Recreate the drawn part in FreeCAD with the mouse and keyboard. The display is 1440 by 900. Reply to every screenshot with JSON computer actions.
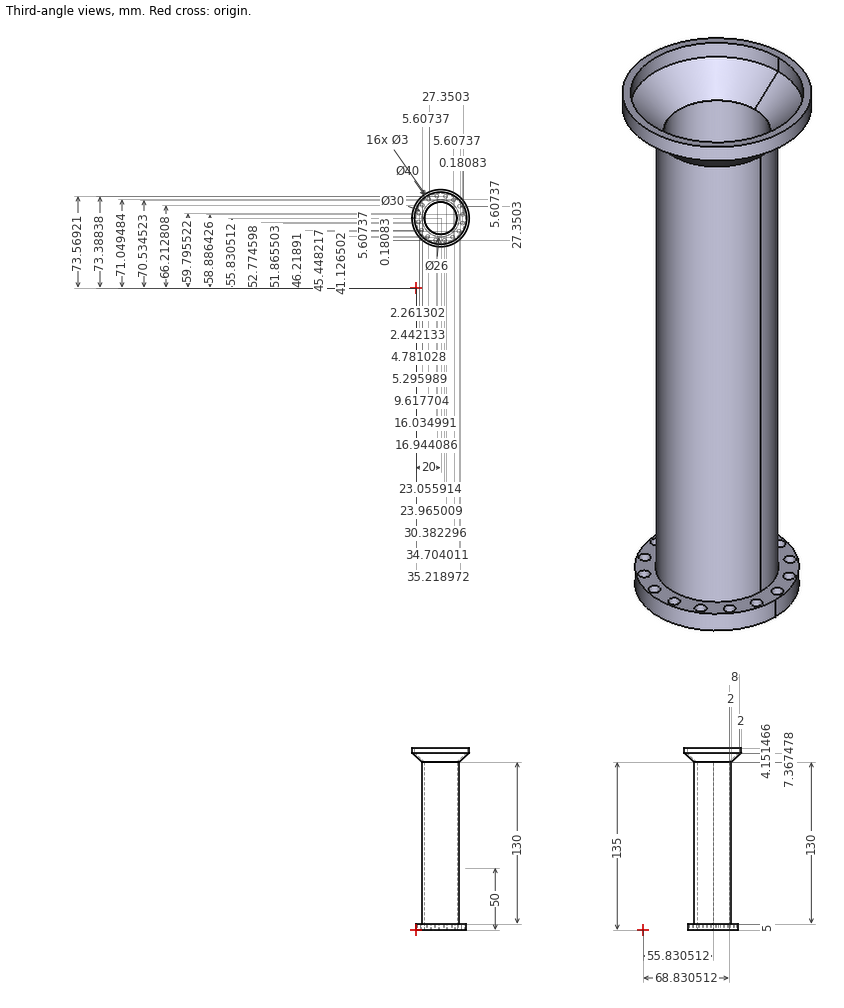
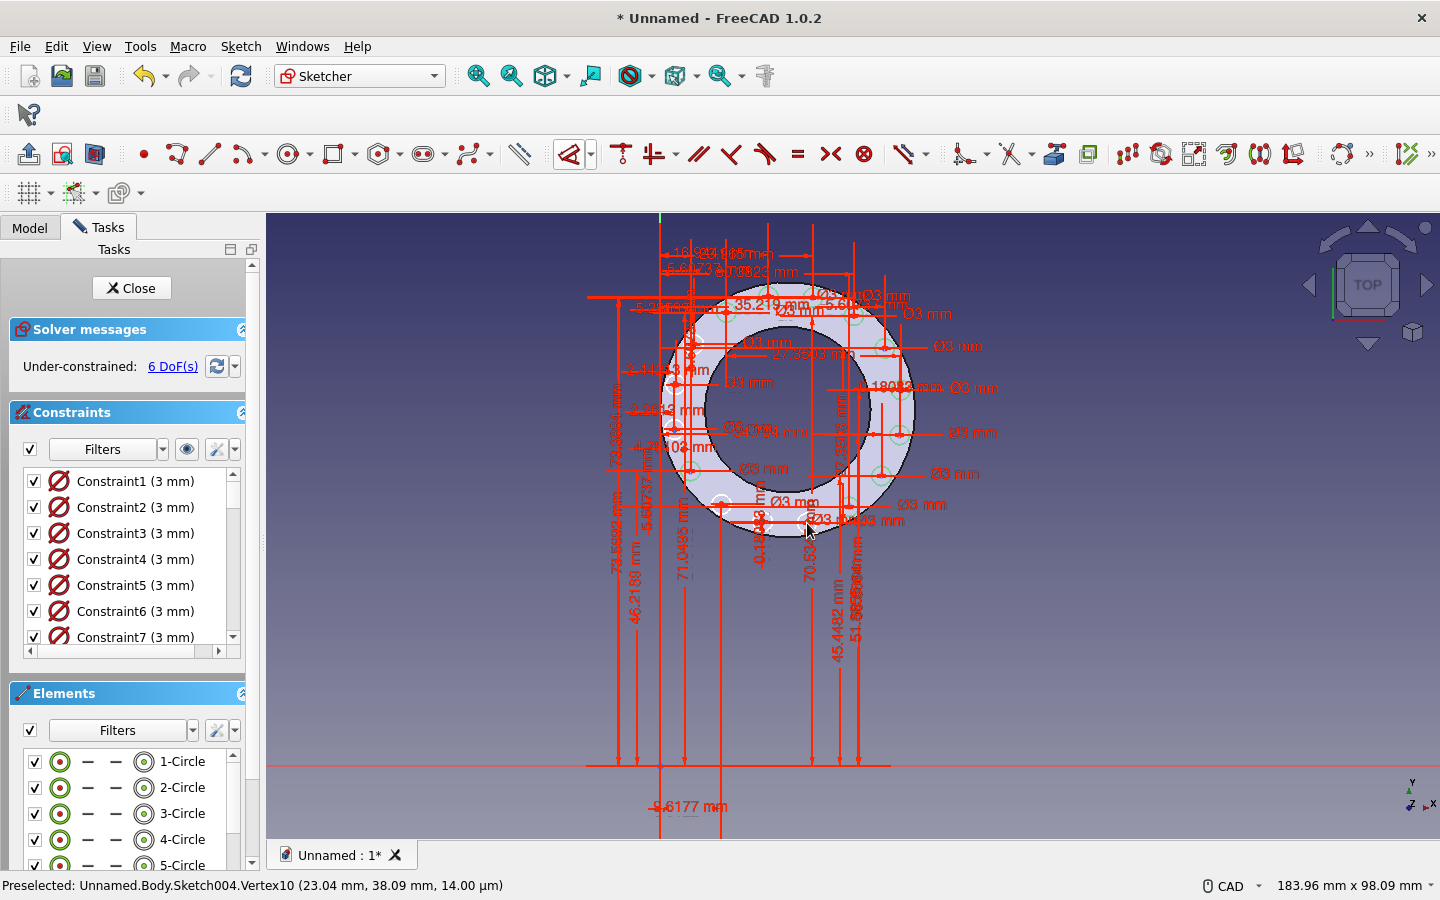
{"action": "key", "text": "l"}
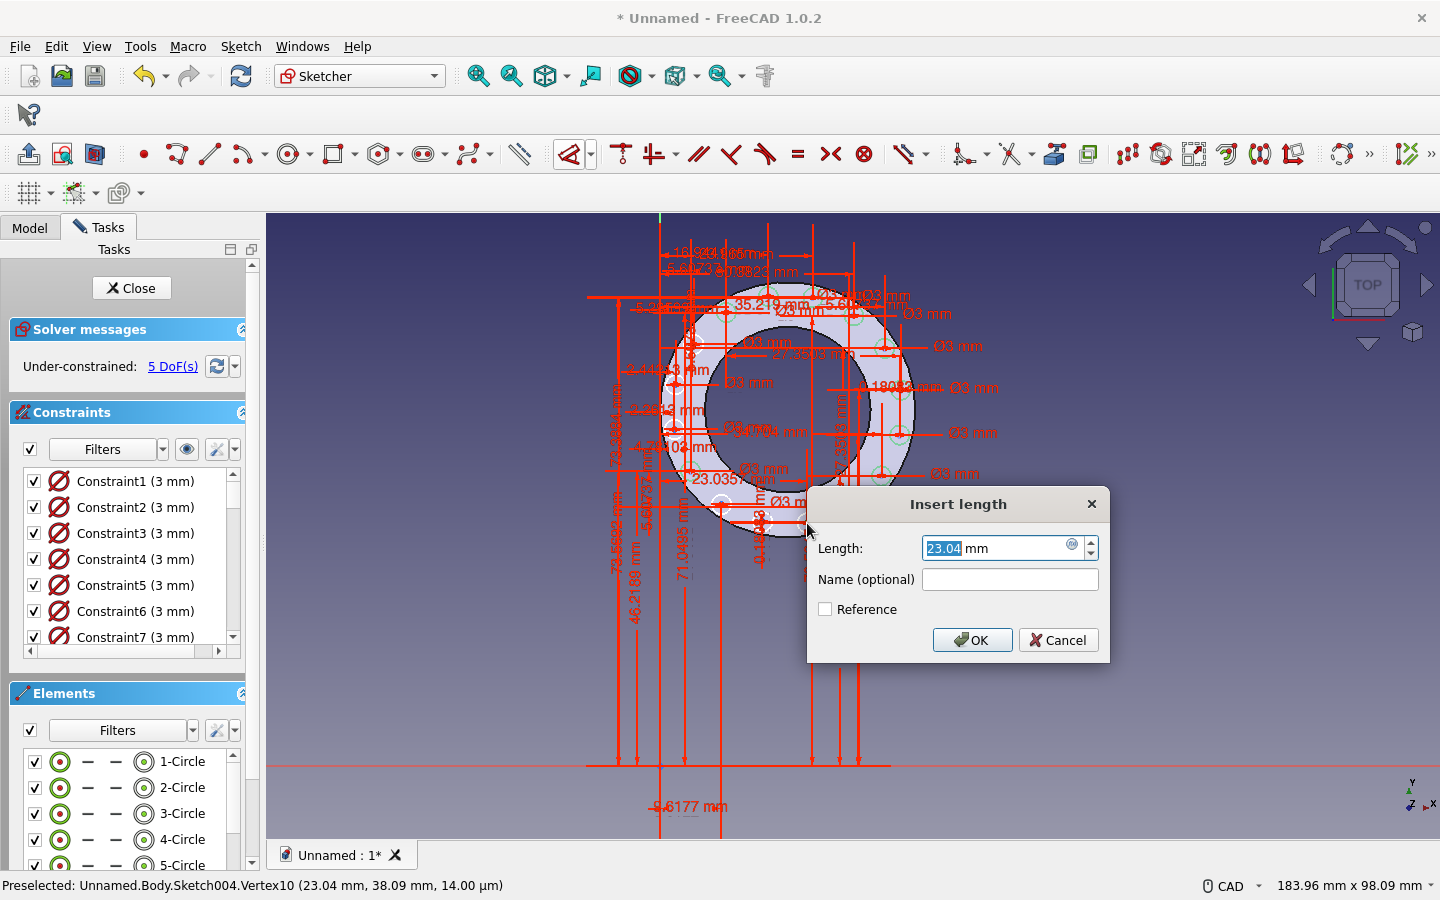
{"action": "type", "text": "23.055914"}
{"action": "key", "text": "Return"}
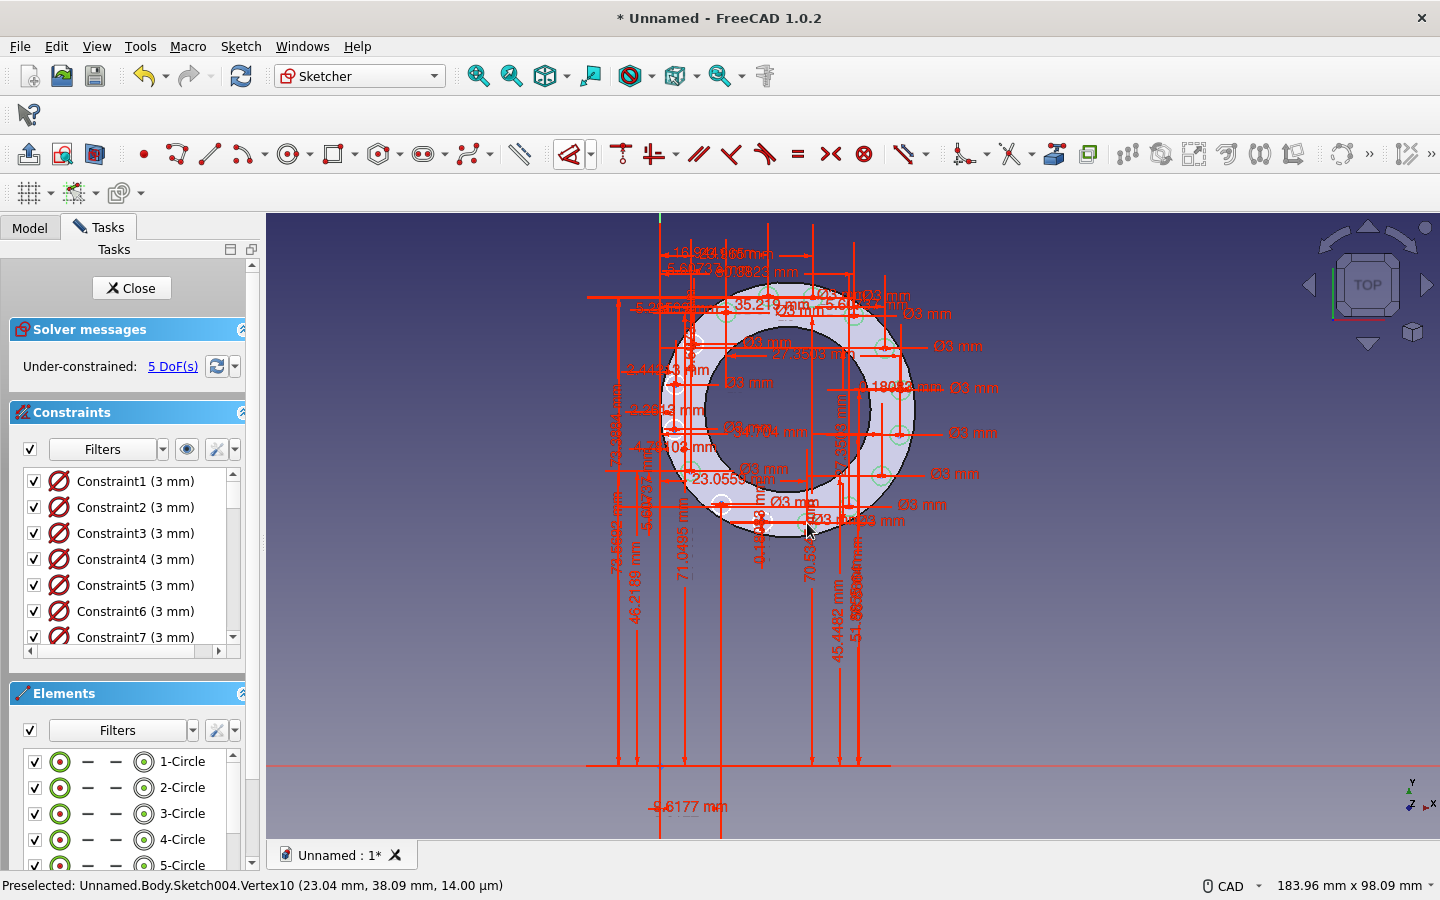
{"action": "left_click", "coordinate": [763, 522]}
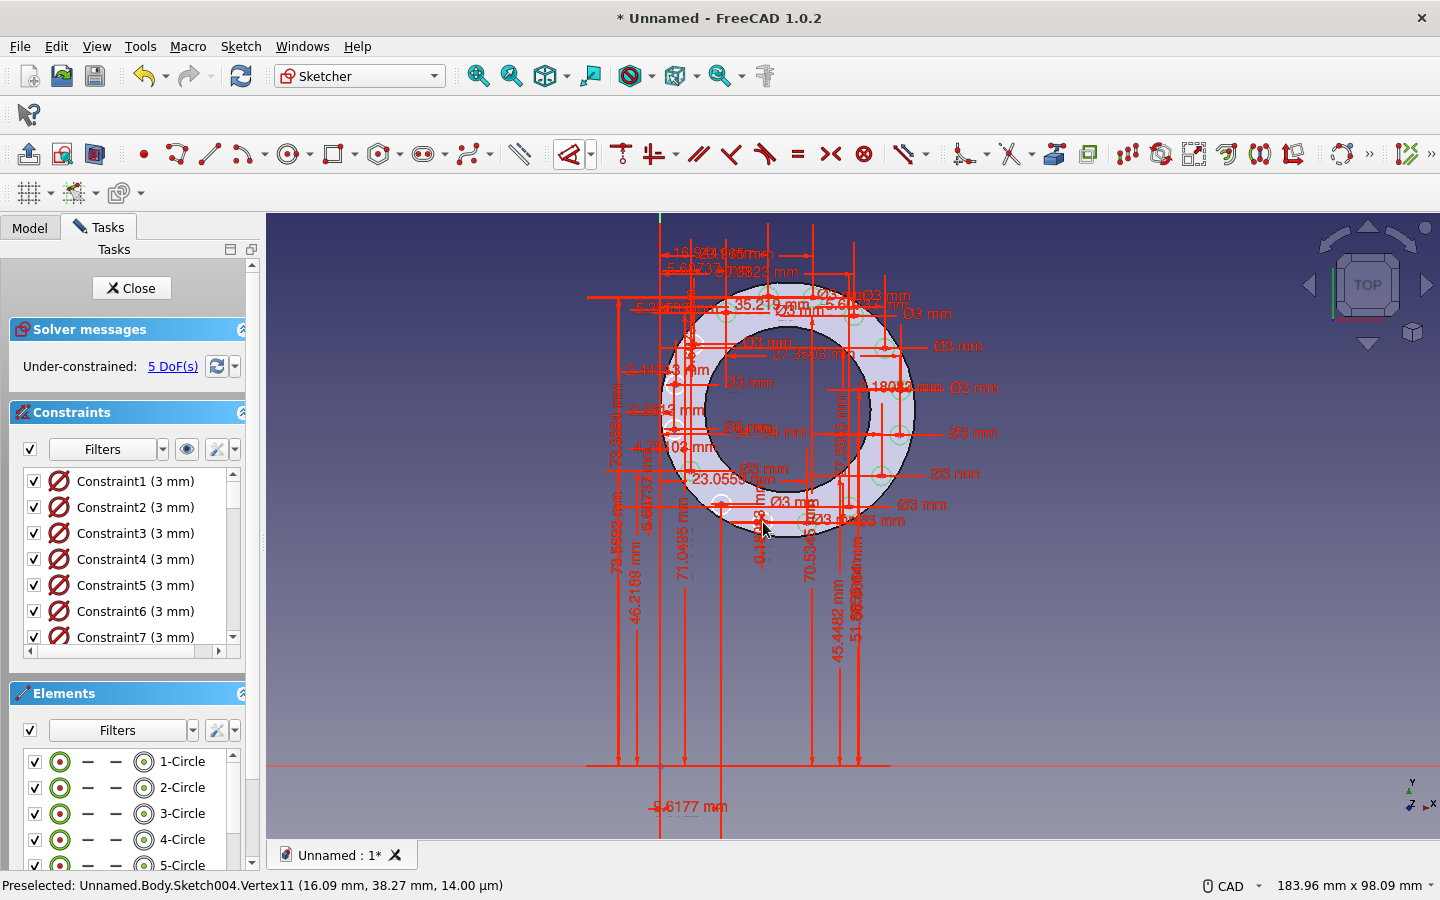
{"action": "key", "text": "l"}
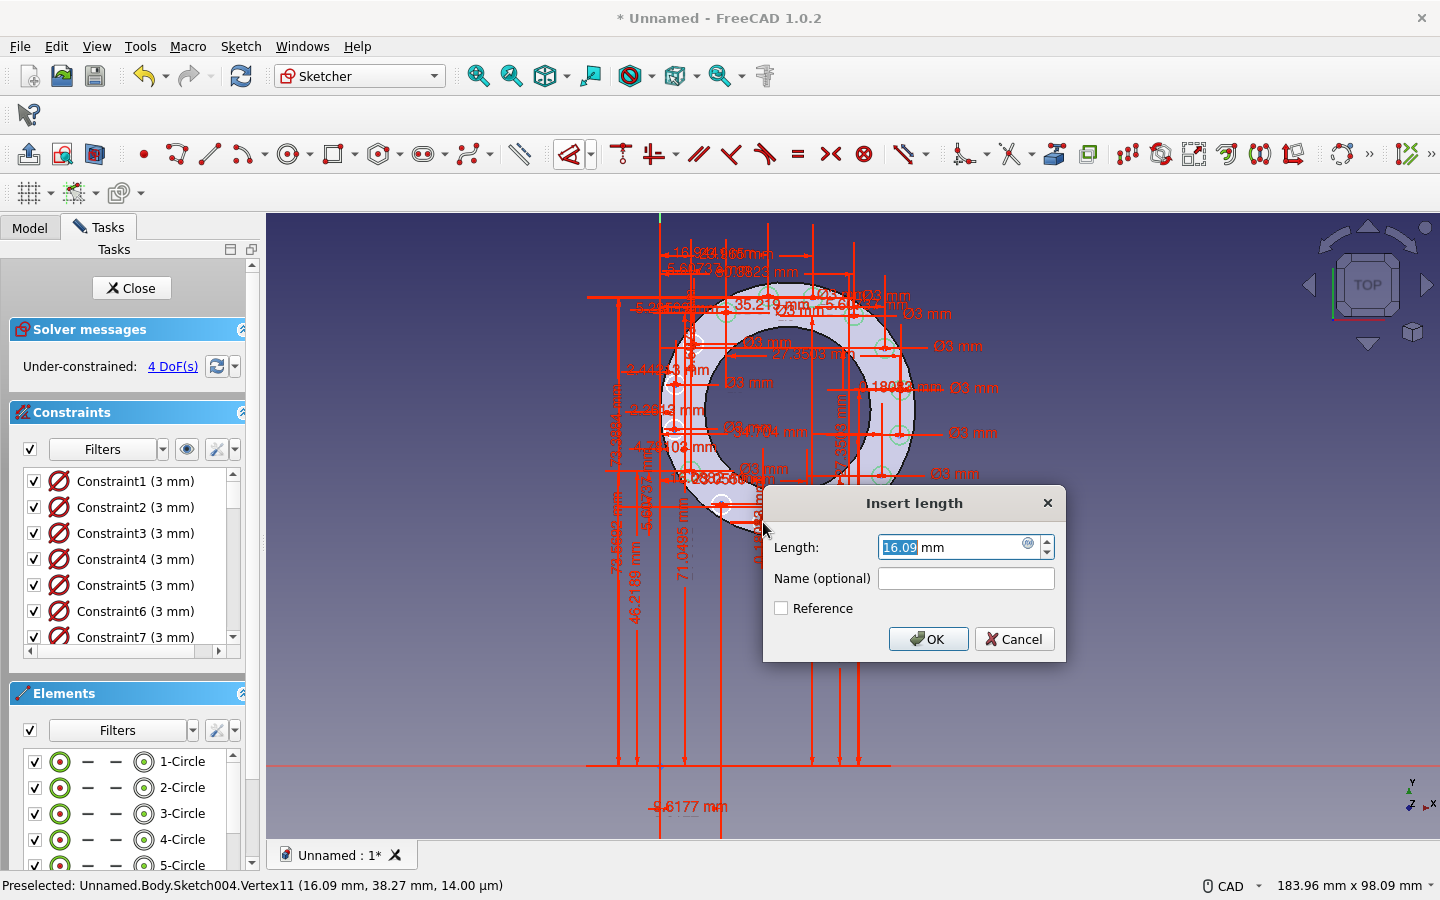
{"action": "type", "text": "16.034991"}
{"action": "key", "text": "Return"}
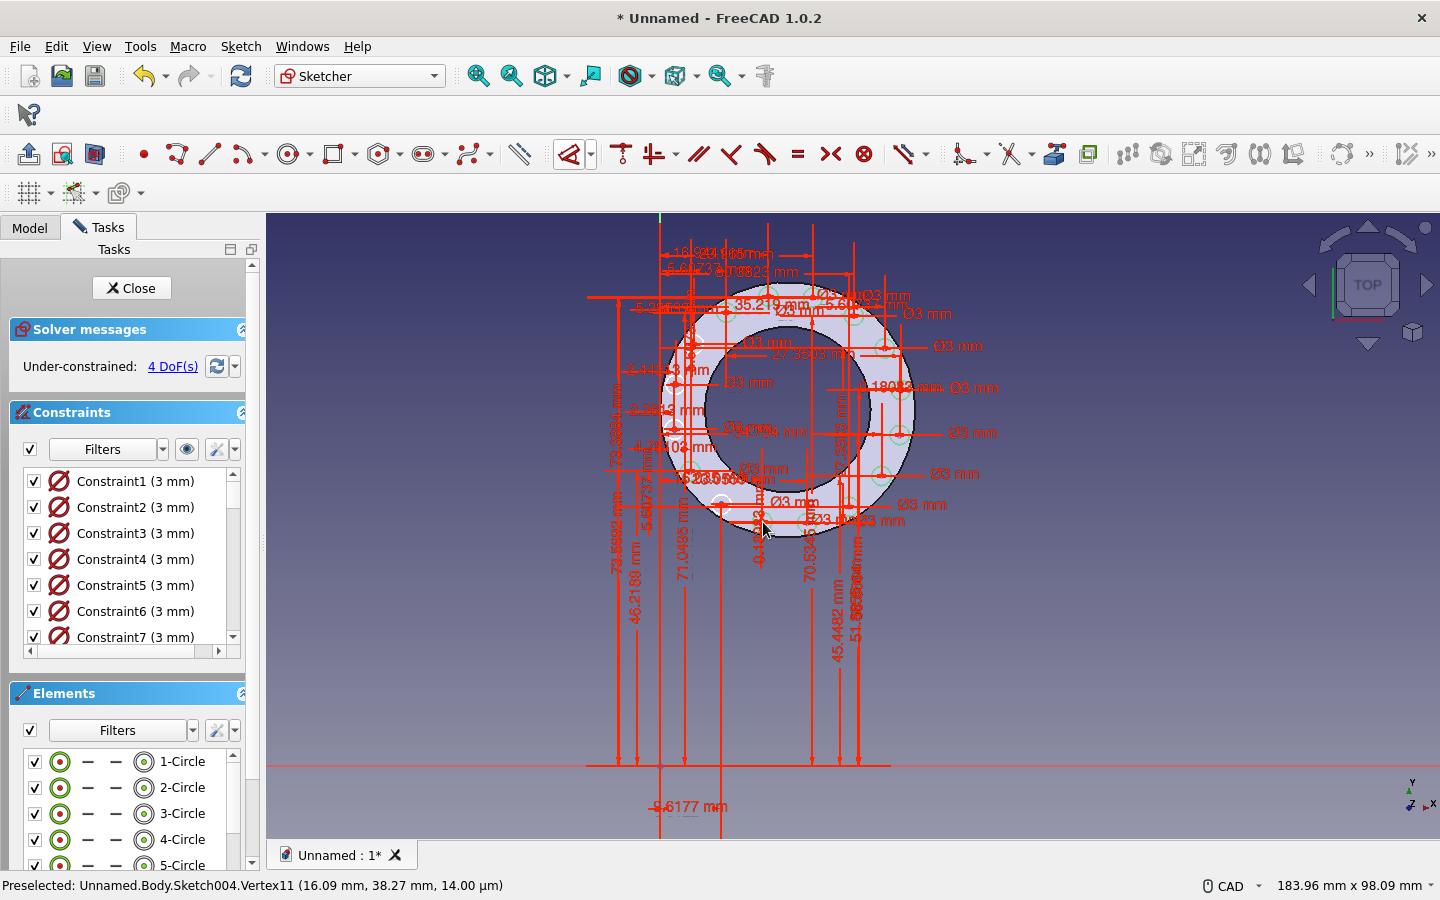
{"action": "left_click", "coordinate": [721, 504]}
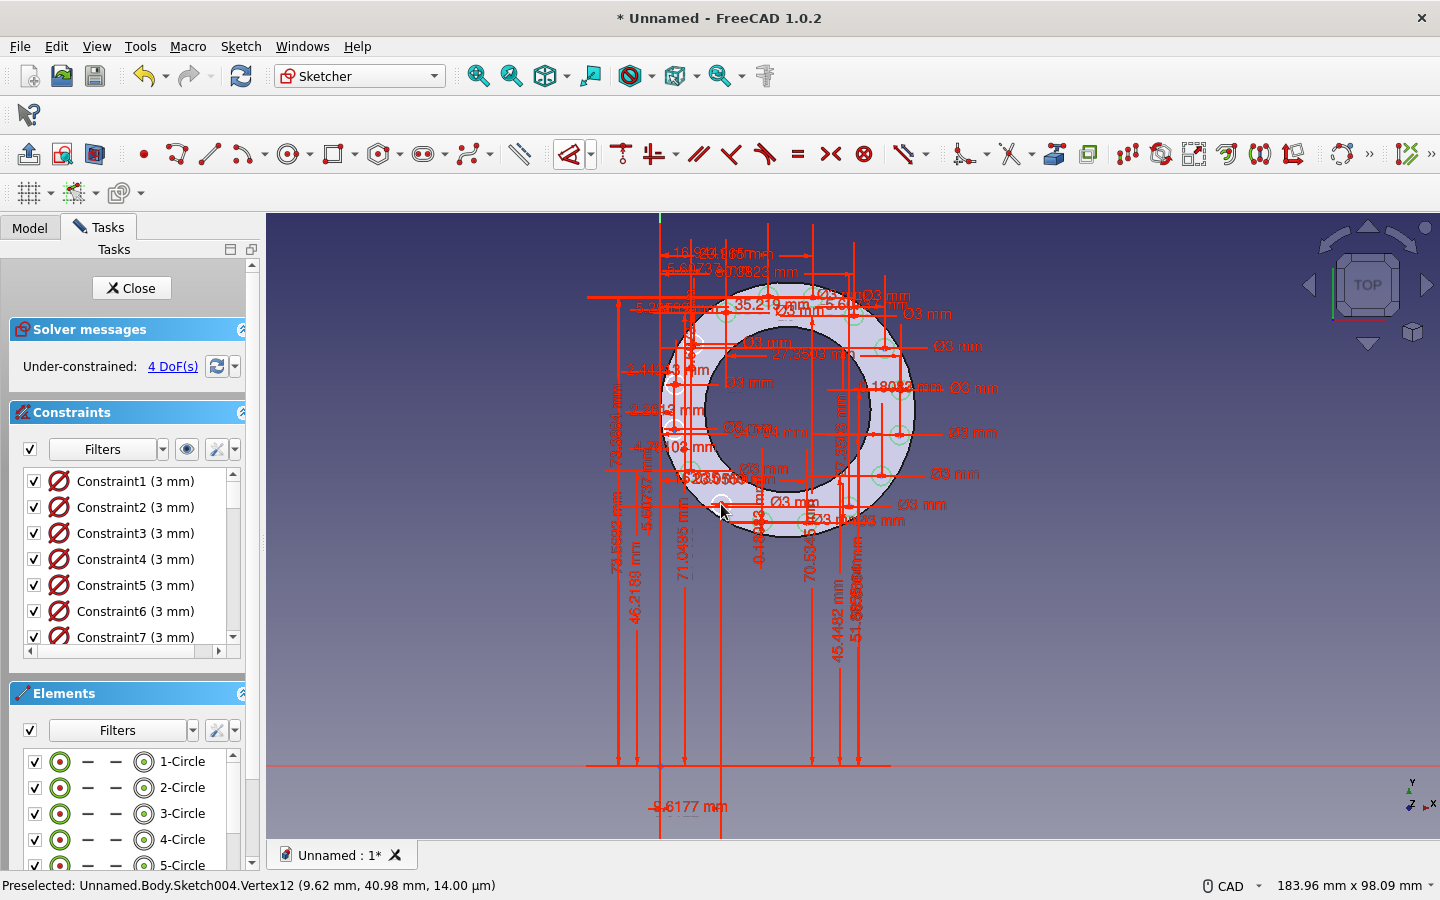
{"action": "left_click", "coordinate": [590, 154]}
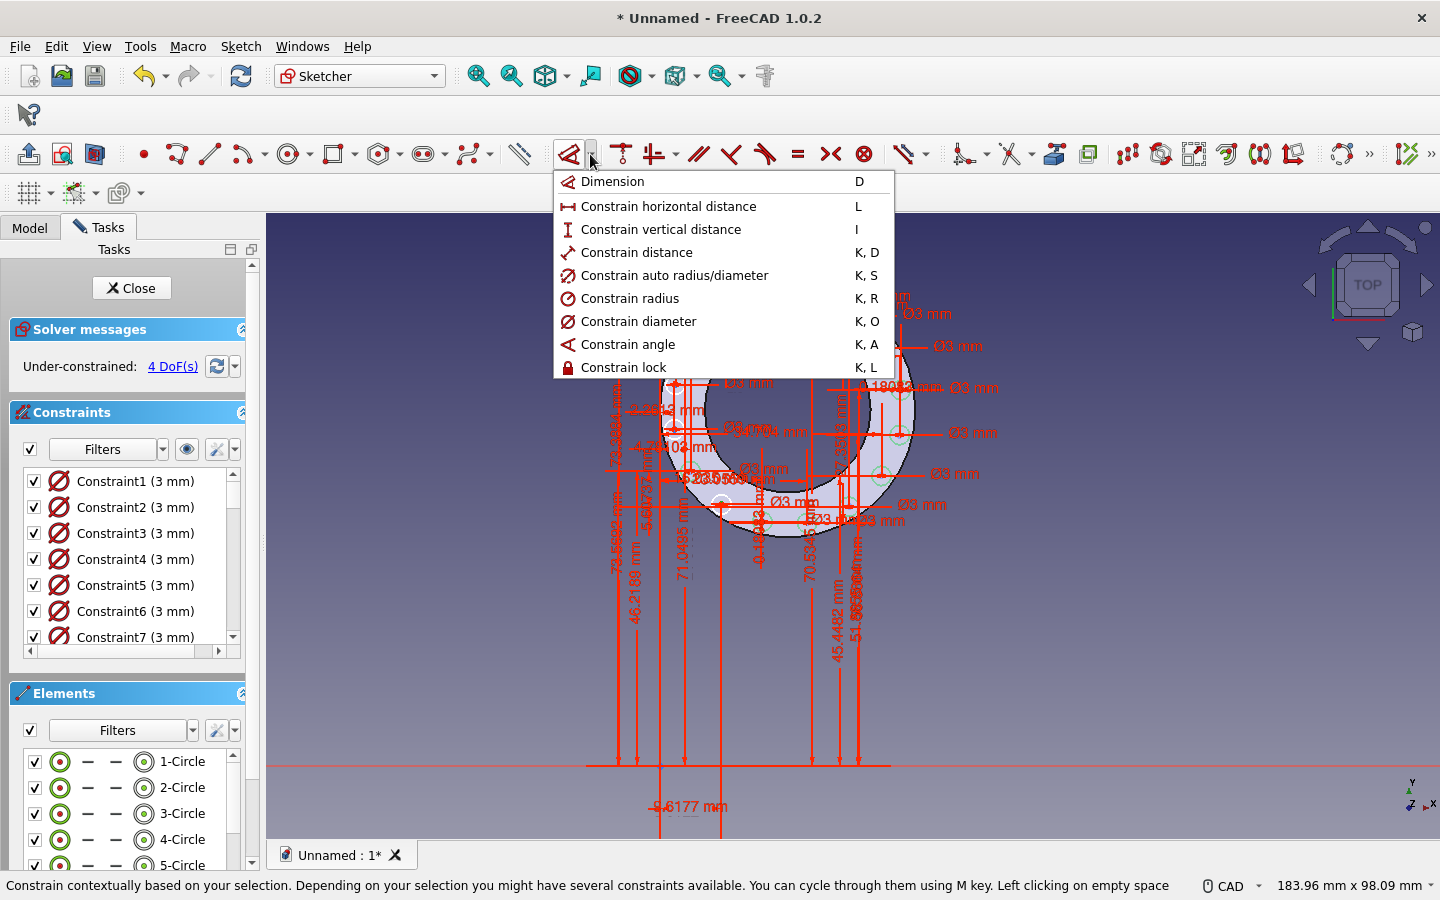
{"action": "left_click", "coordinate": [724, 230]}